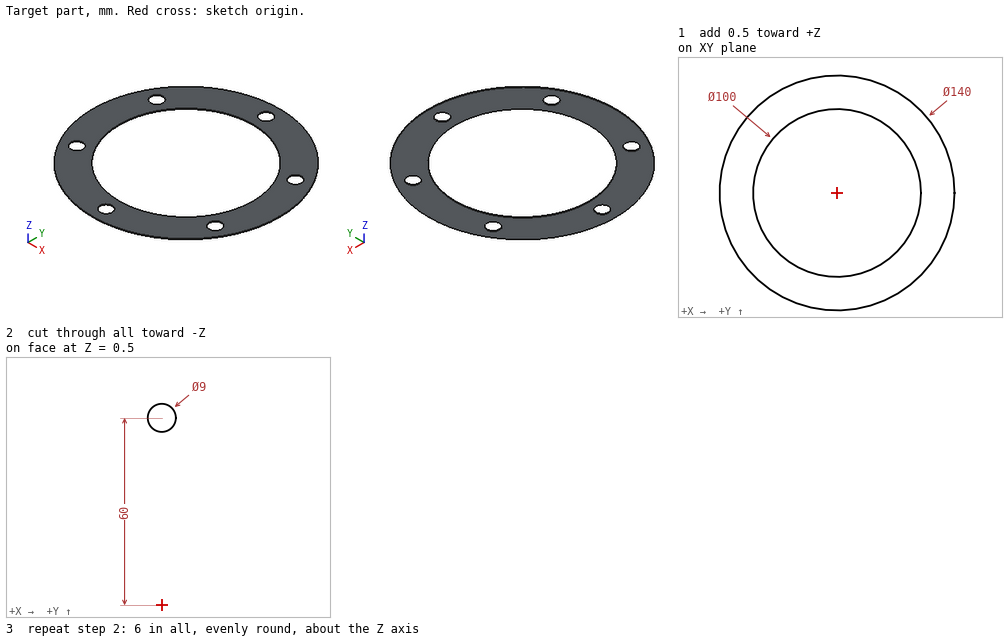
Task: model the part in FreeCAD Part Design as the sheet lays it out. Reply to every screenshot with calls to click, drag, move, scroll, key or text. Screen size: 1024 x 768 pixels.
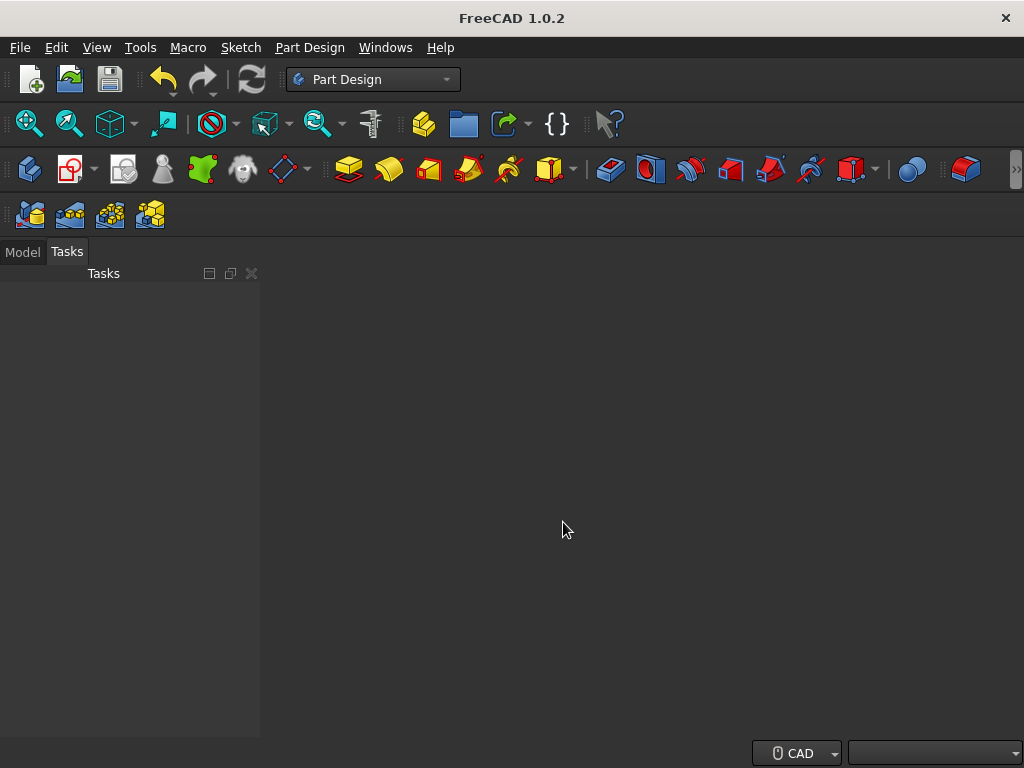
click(30, 80)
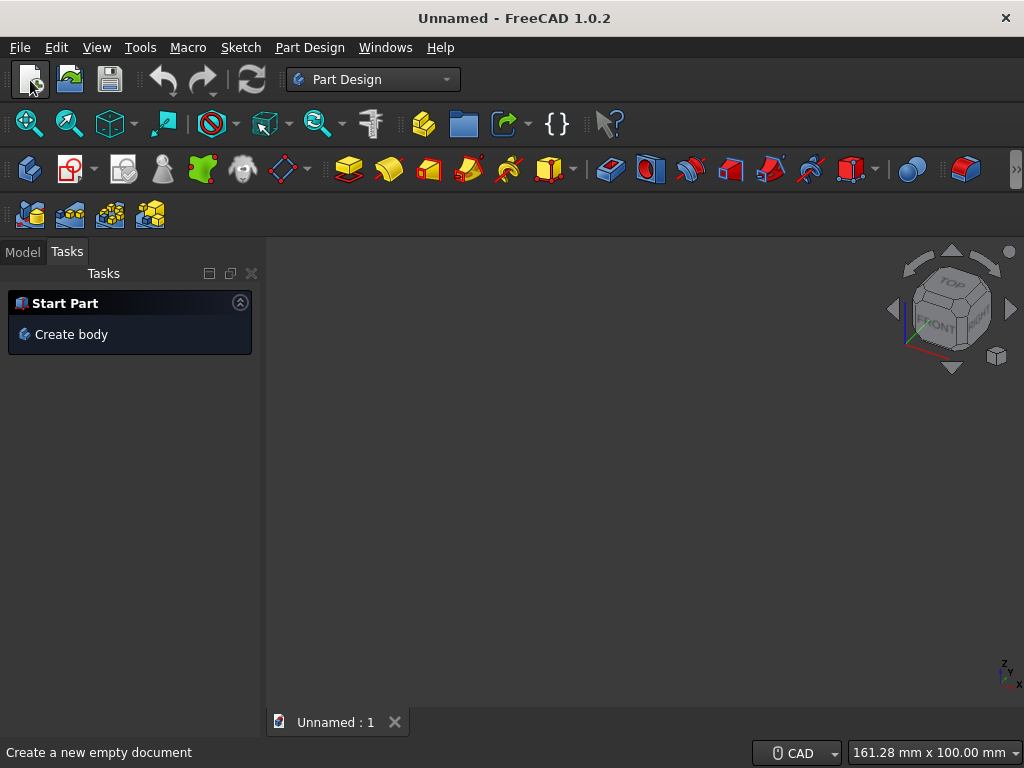
click(70, 170)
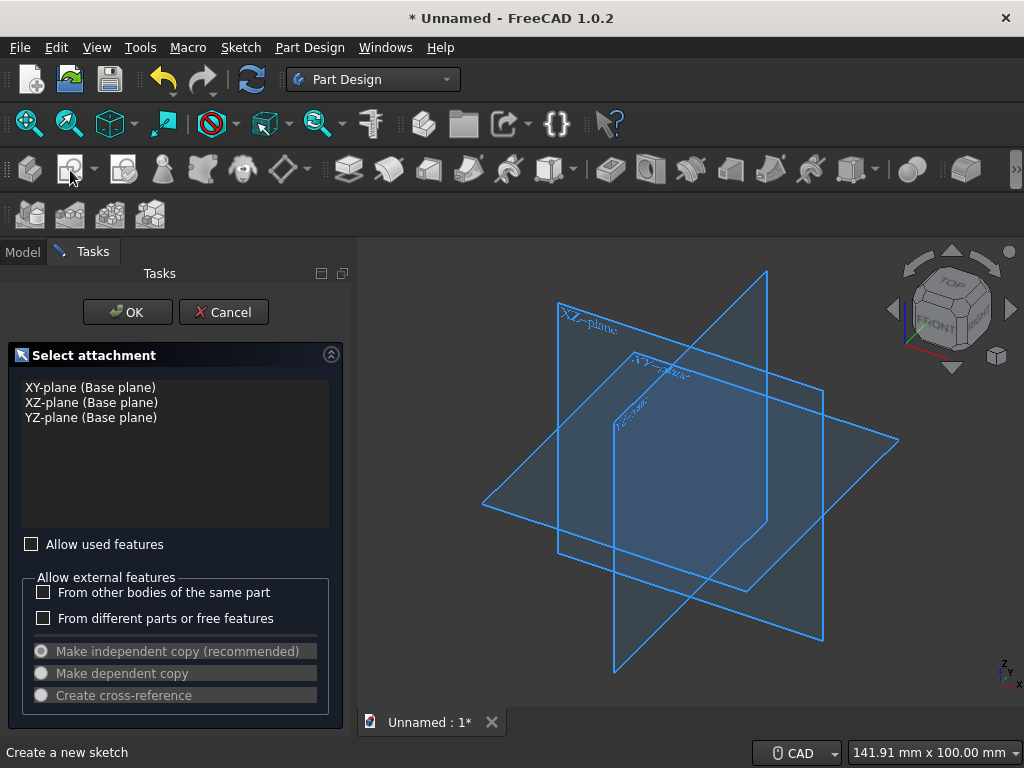
click(82, 388)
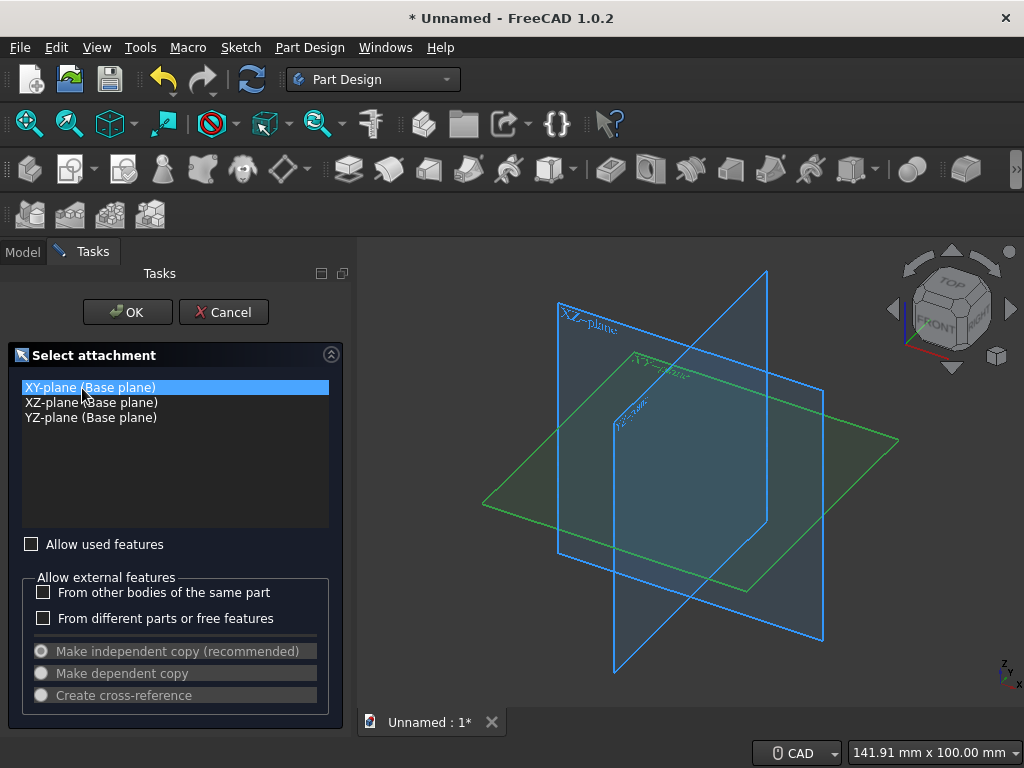
click(128, 312)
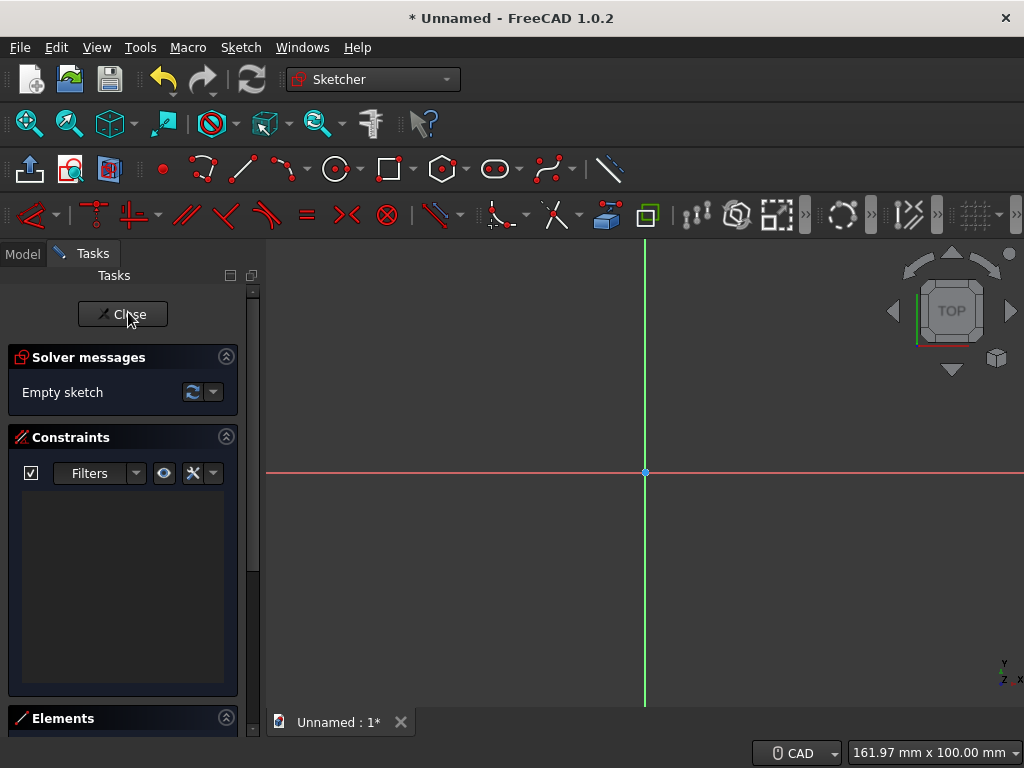
scroll(521, 473, down, 4)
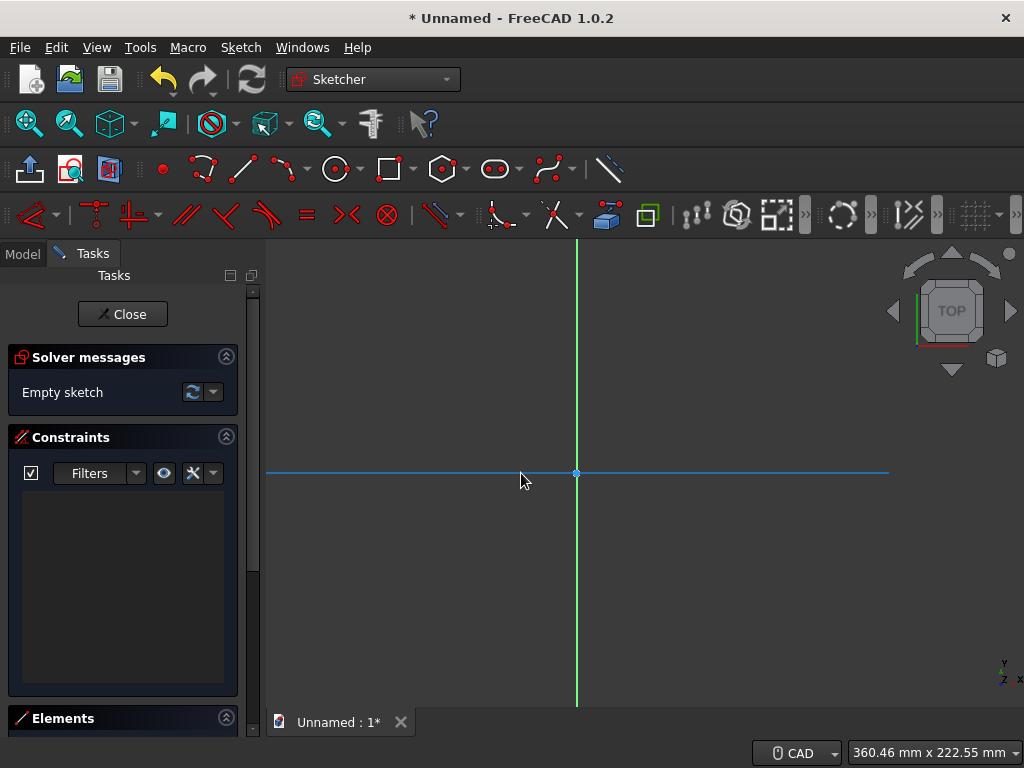
click(336, 170)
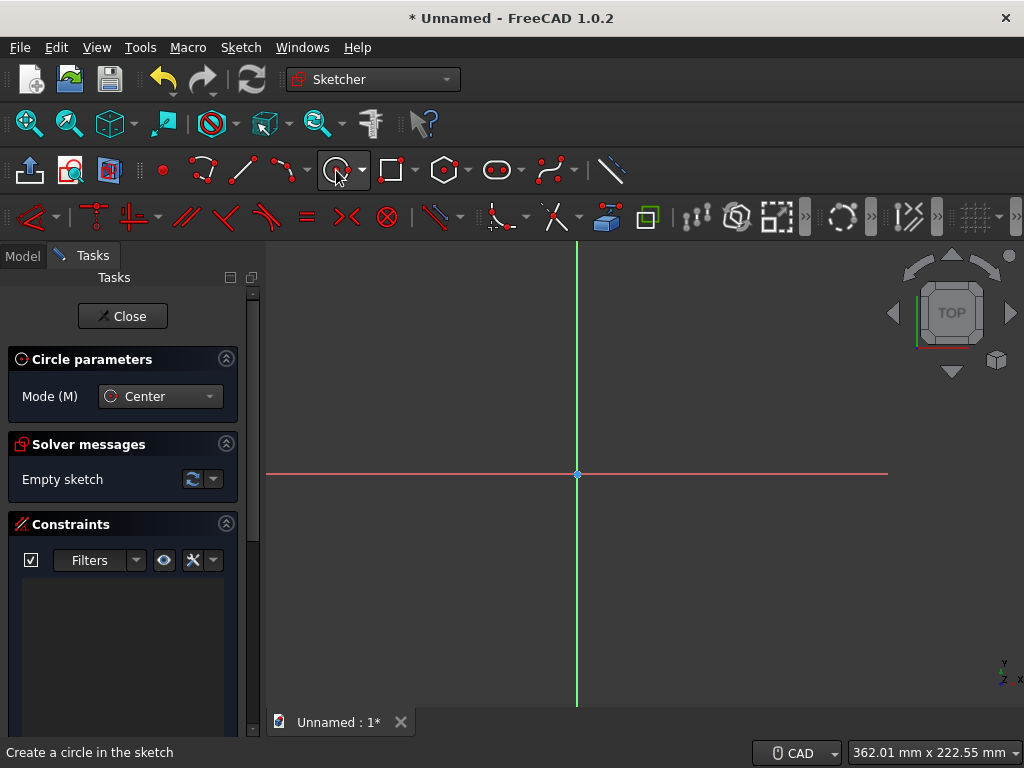
click(577, 474)
move(681, 371)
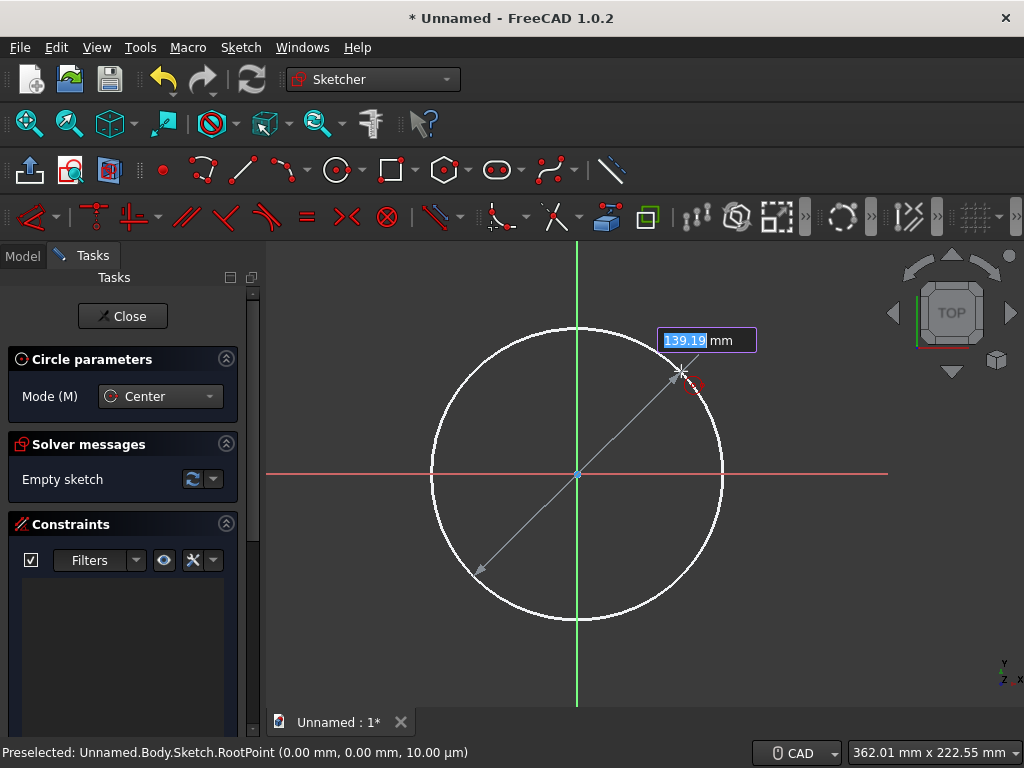
text(140)
key(Return)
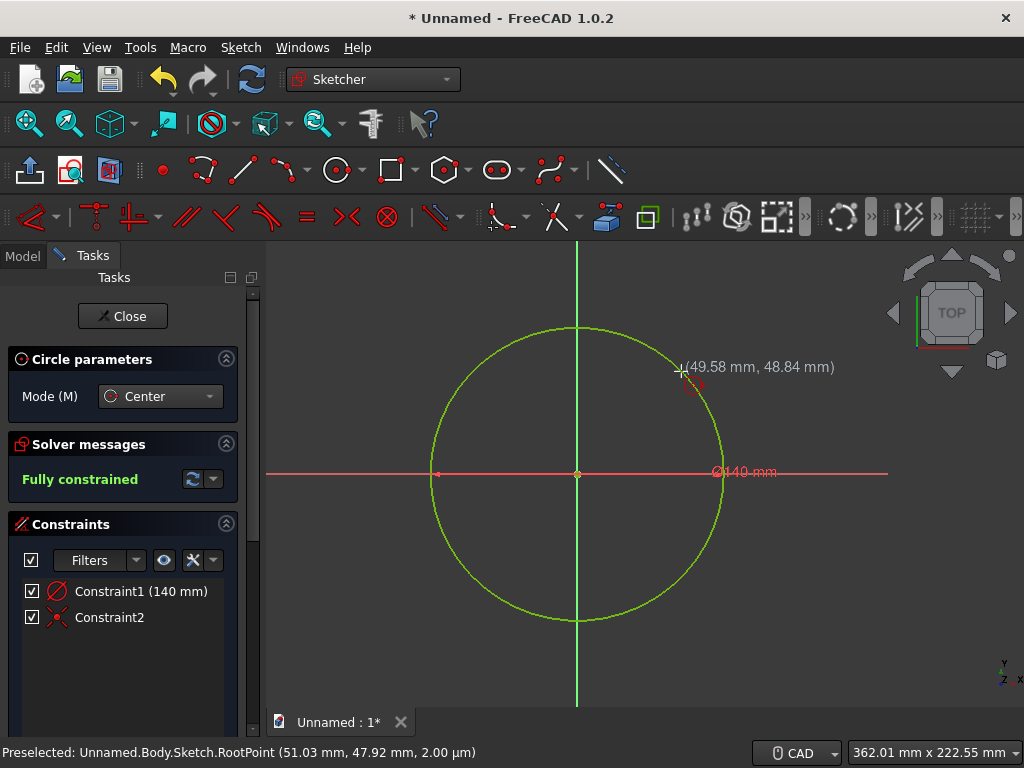
click(577, 474)
move(651, 400)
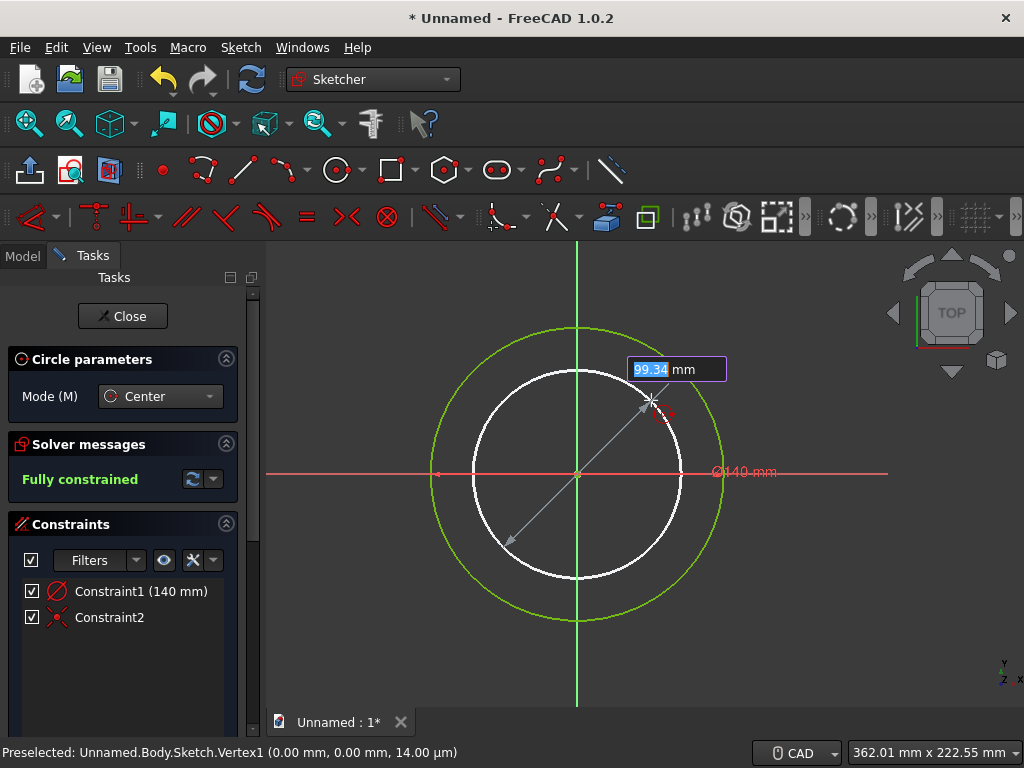
text(100)
key(Return)
key(Escape)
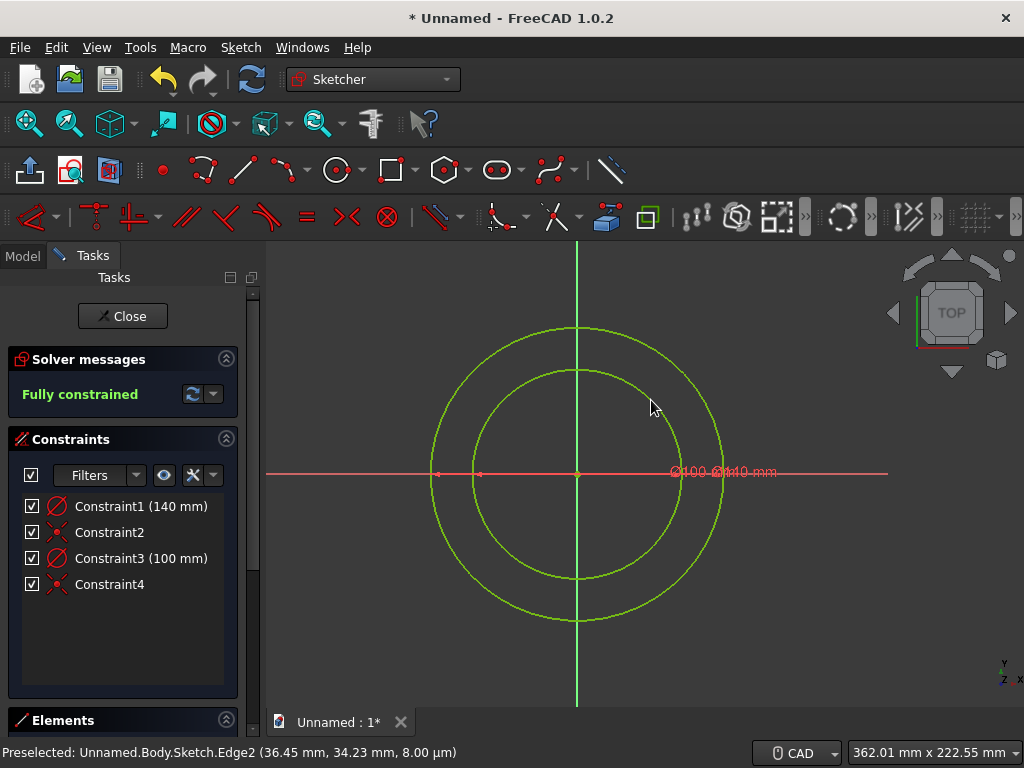
click(123, 316)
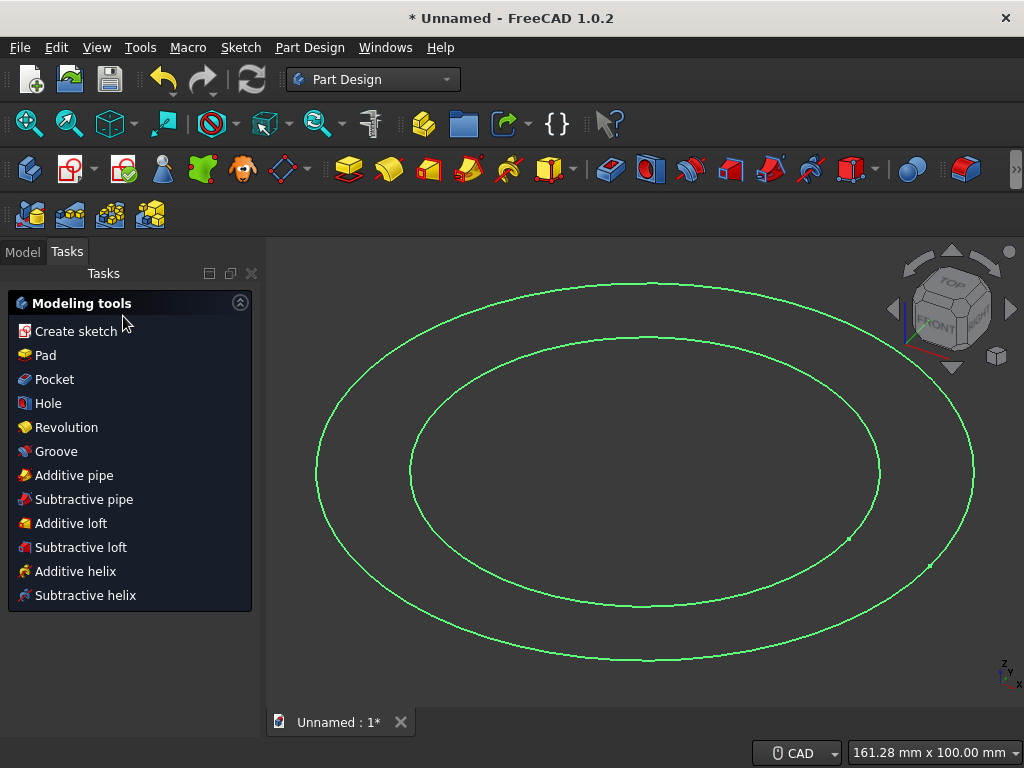
click(350, 170)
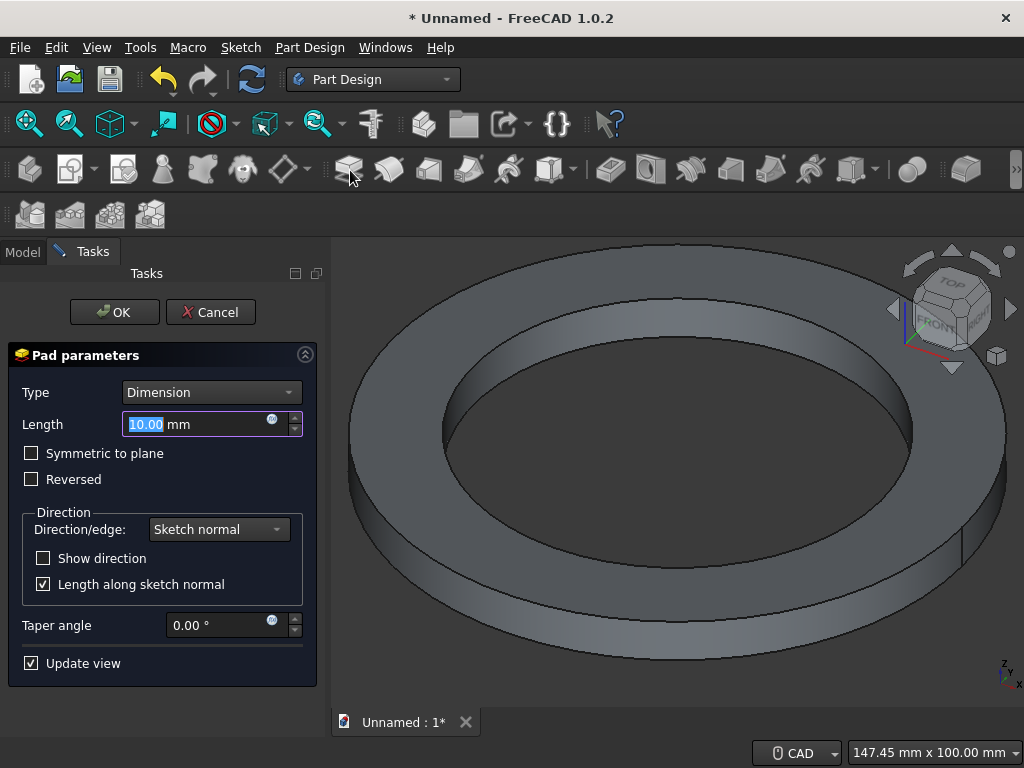
text(0.5)
key(Tab)